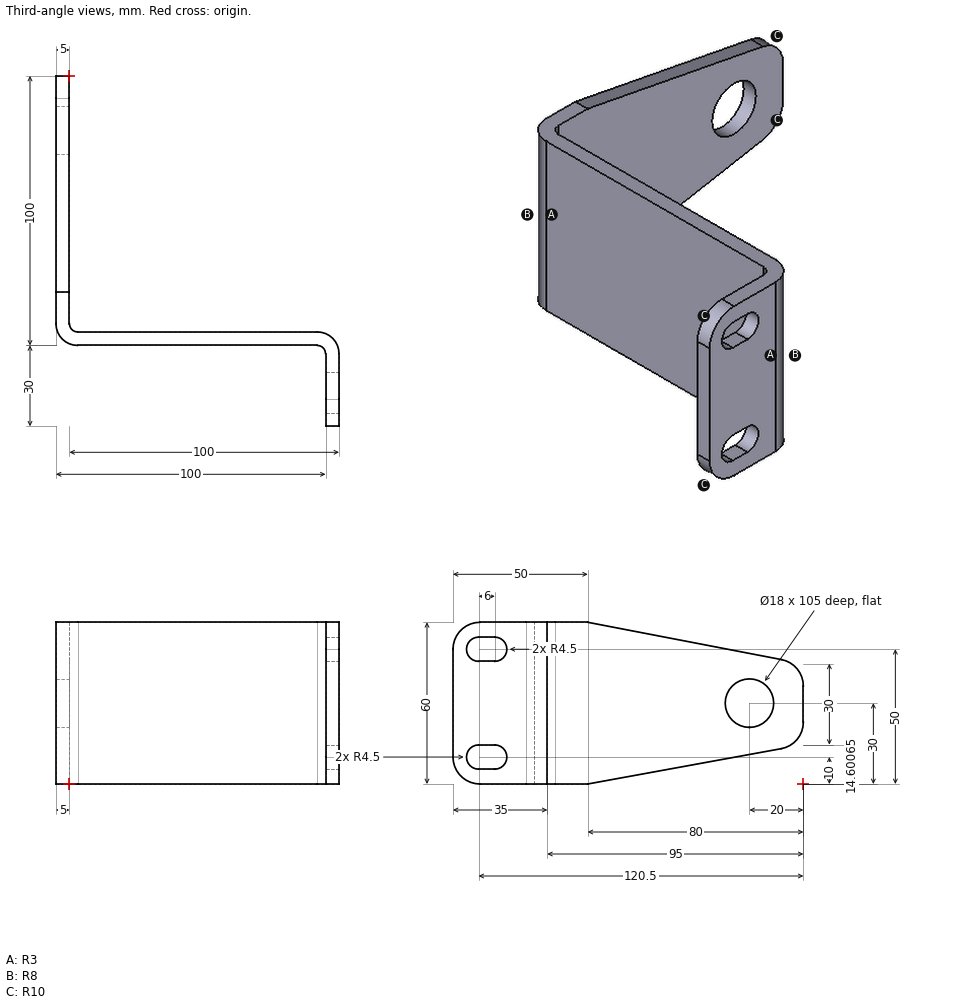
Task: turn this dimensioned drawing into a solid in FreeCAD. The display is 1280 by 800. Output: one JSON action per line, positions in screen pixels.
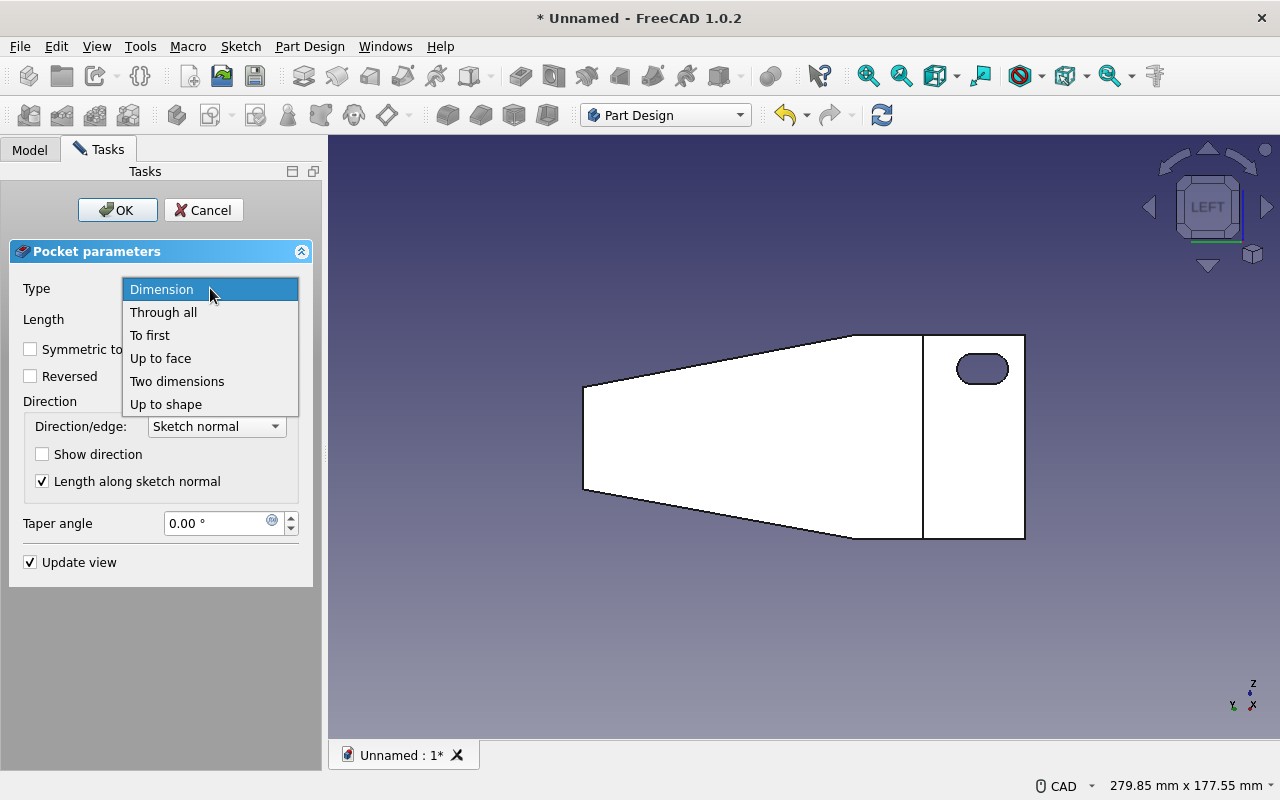
{"action": "left_click", "coordinate": [208, 312]}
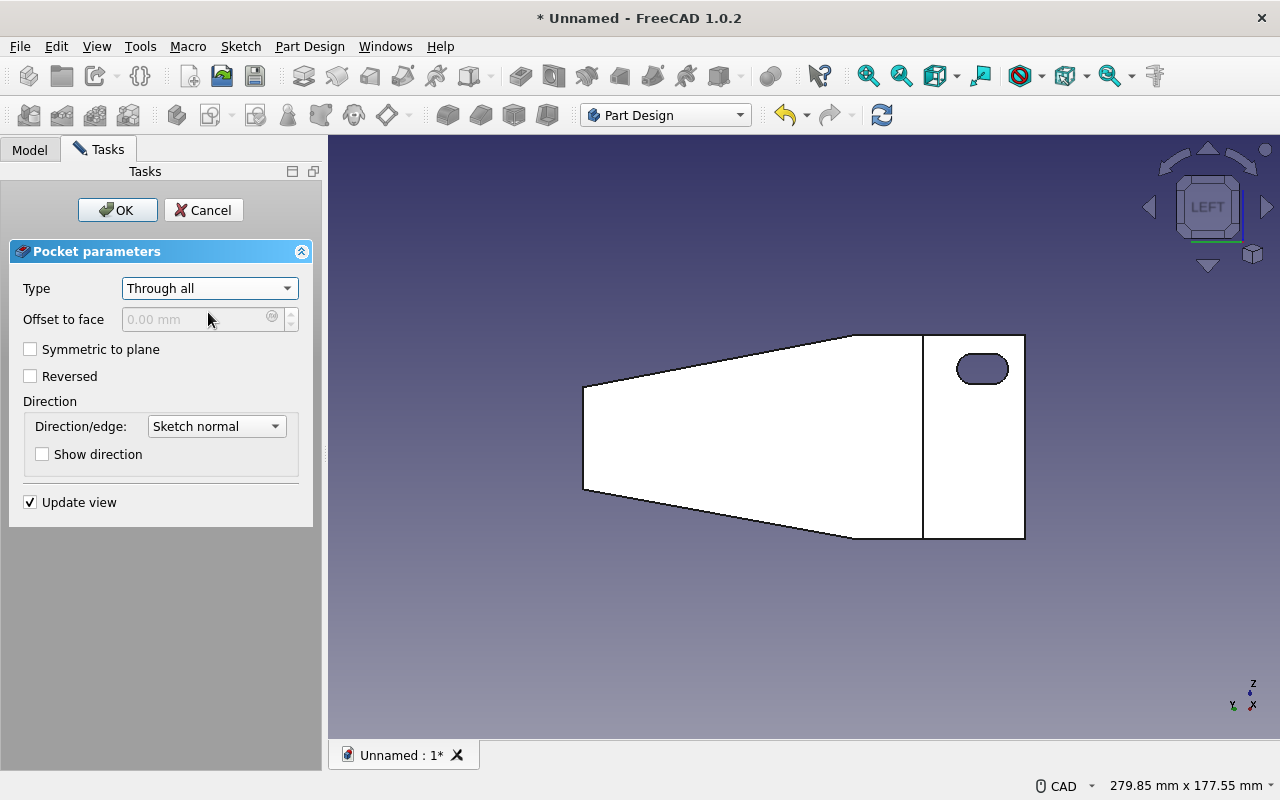
{"action": "left_click", "coordinate": [118, 210]}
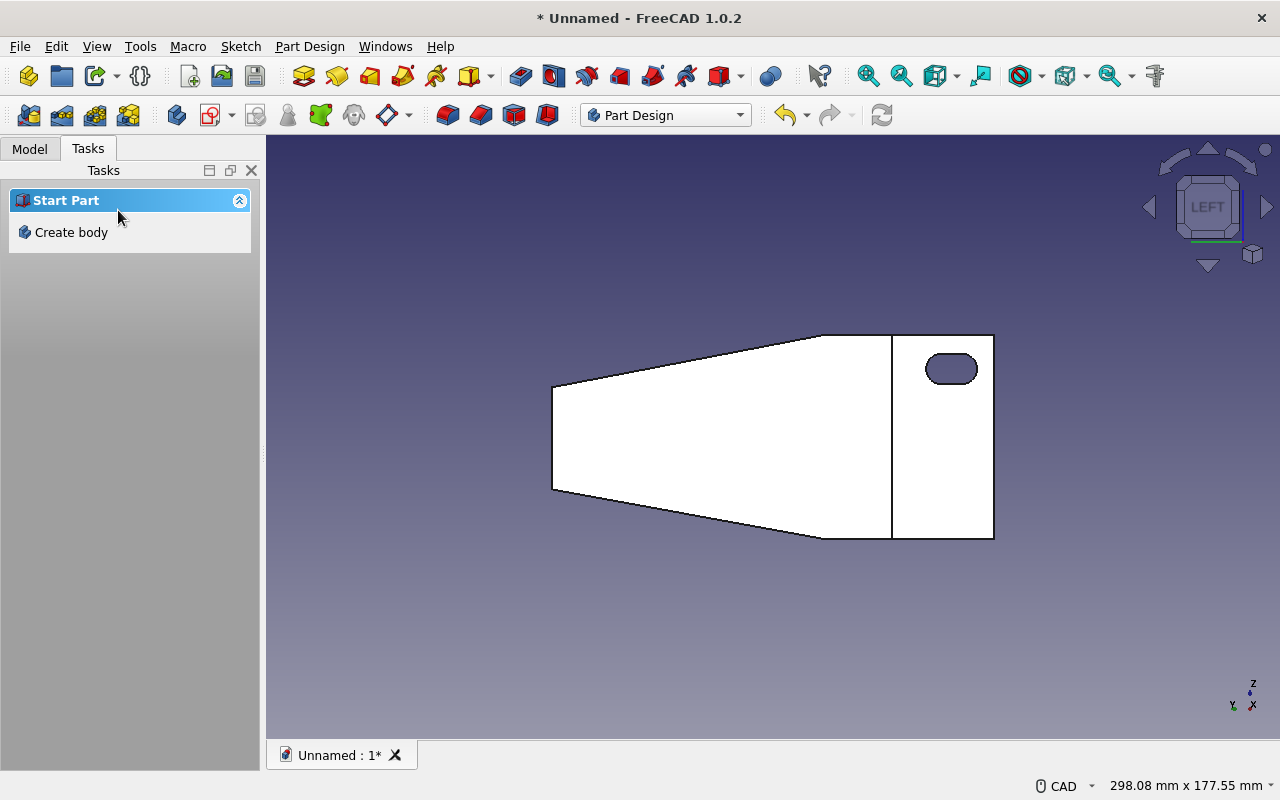
{"action": "left_click", "coordinate": [869, 76]}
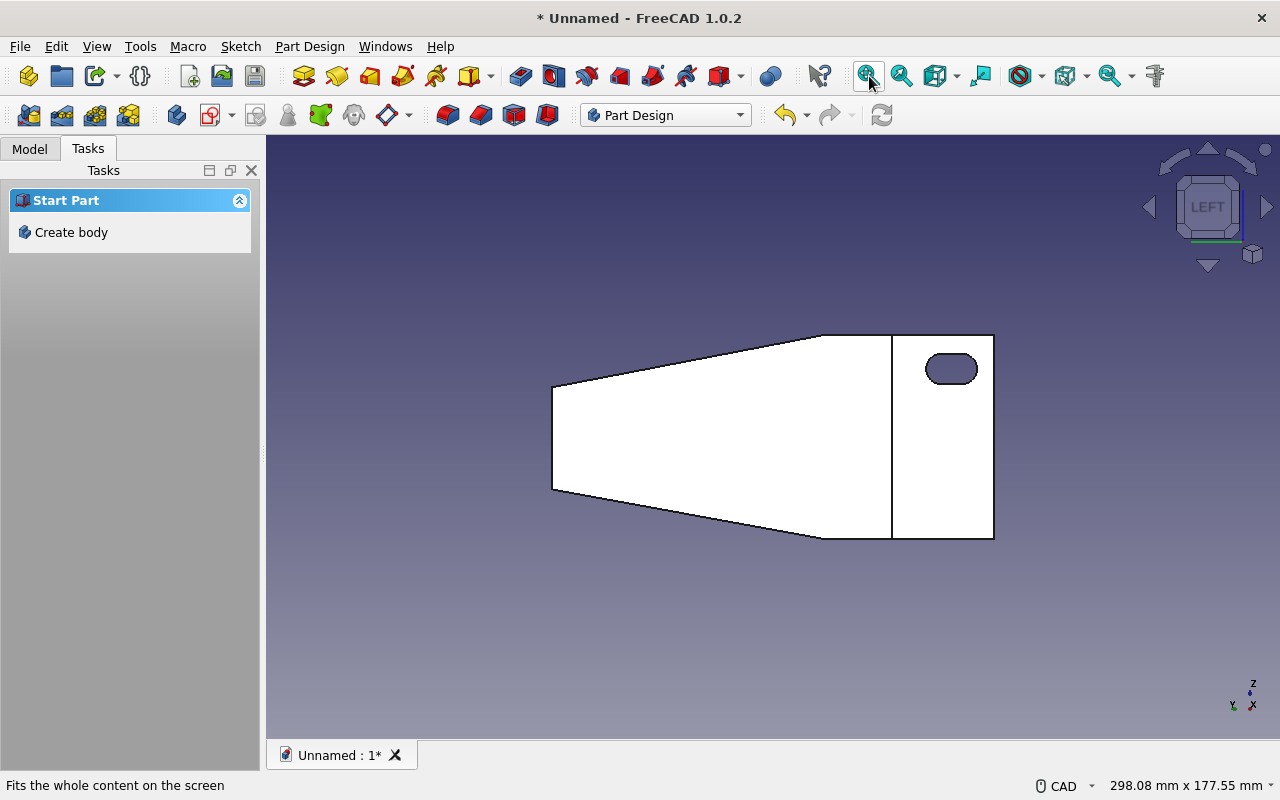
{"action": "key", "text": "0"}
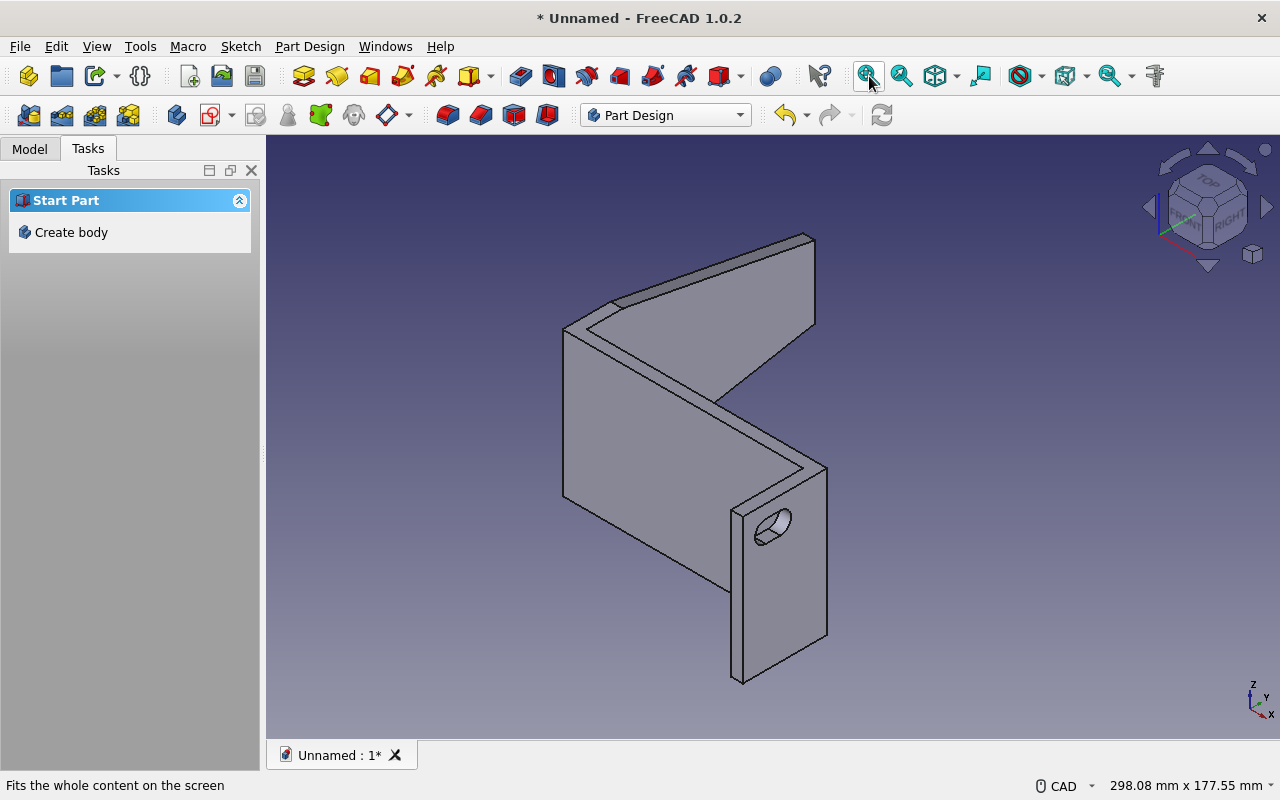
{"action": "left_click", "coordinate": [785, 599]}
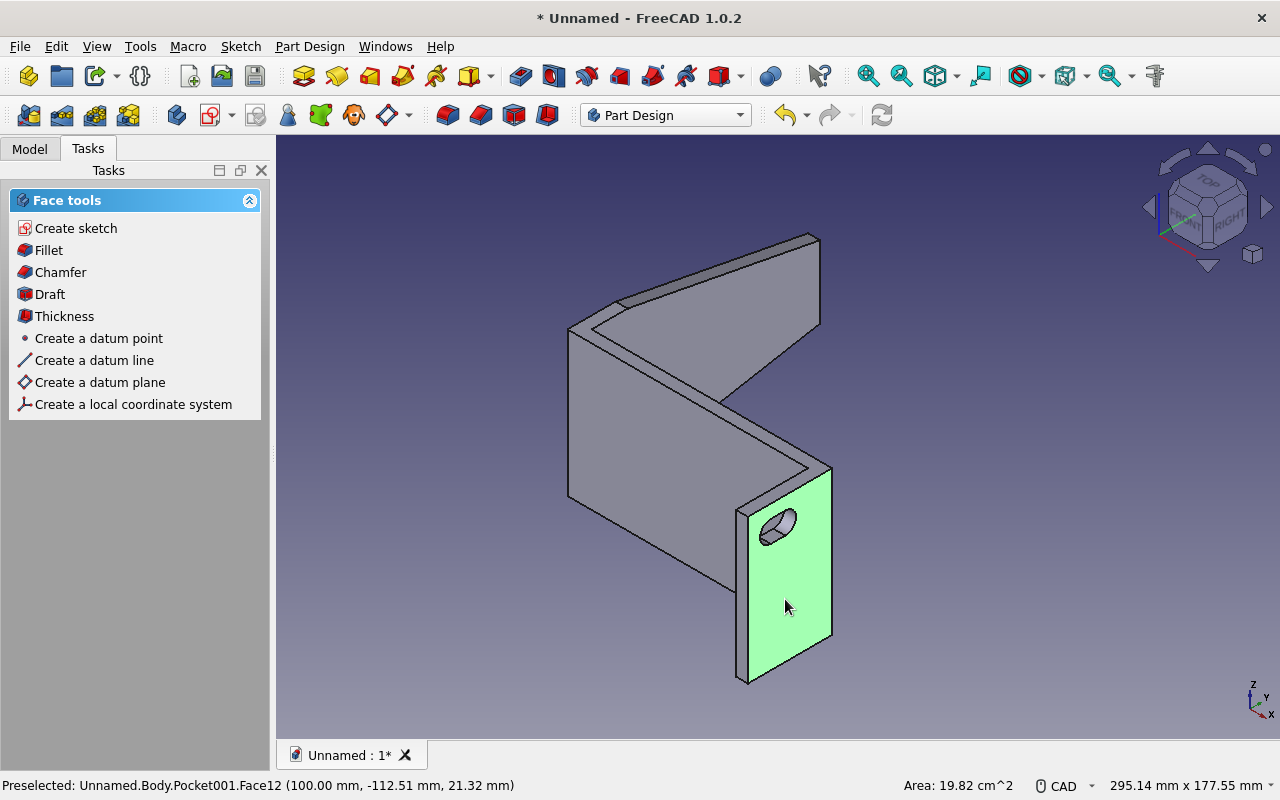
{"action": "left_click", "coordinate": [210, 116]}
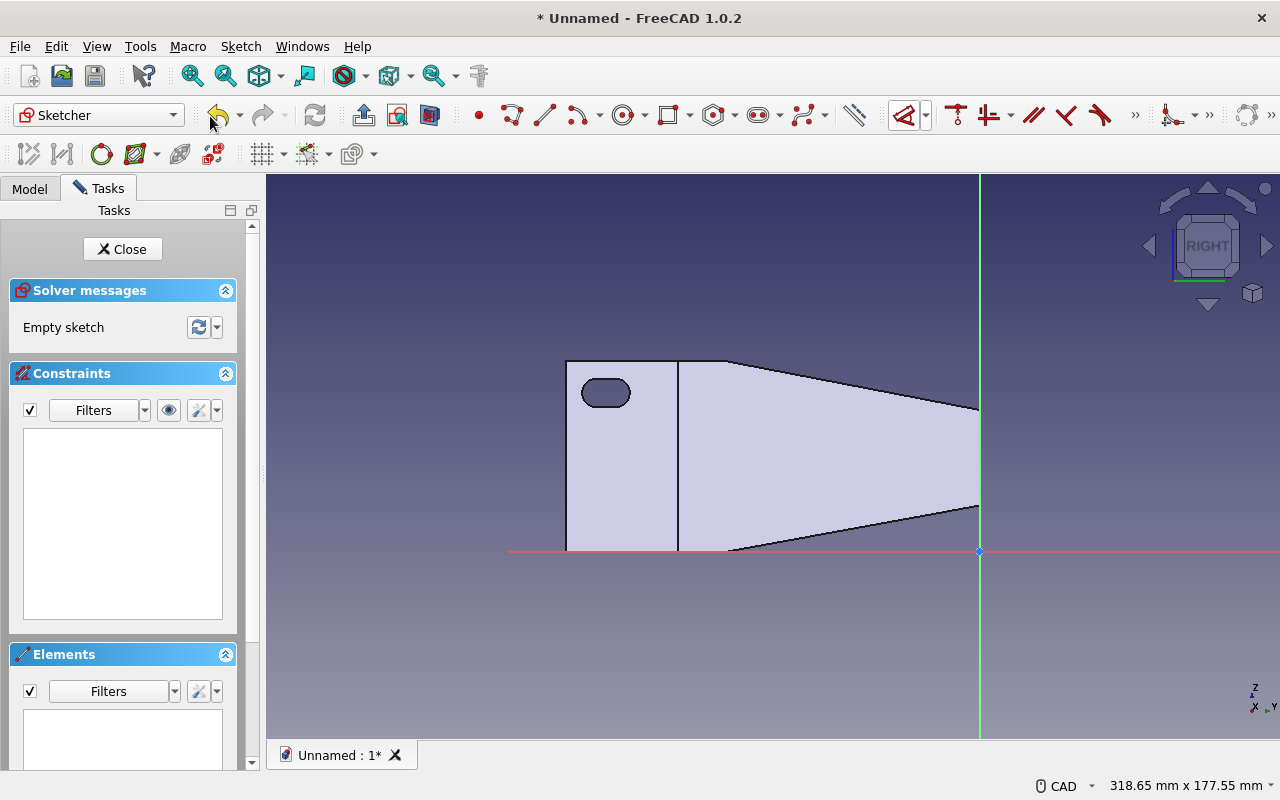
{"action": "scroll", "coordinate": [596, 526], "scroll_direction": "up", "scroll_amount": 12}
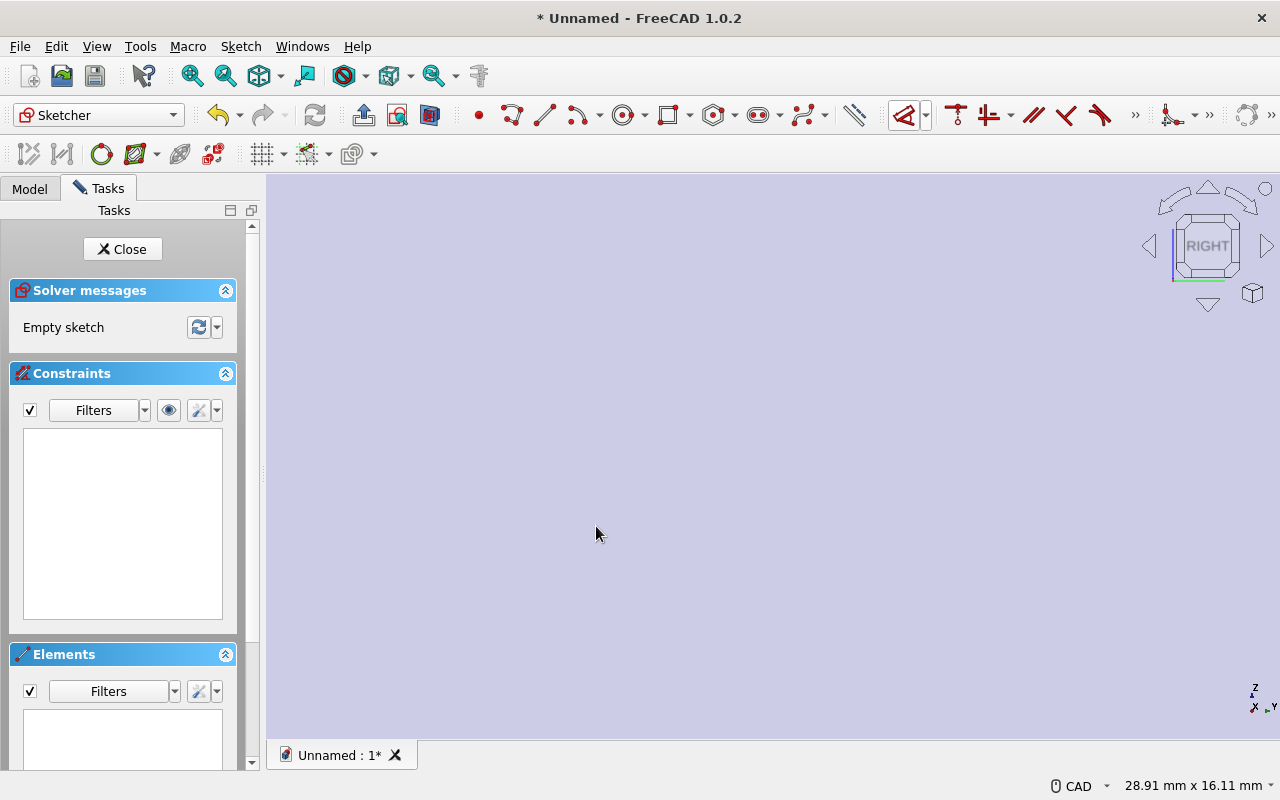
{"action": "left_click", "coordinate": [758, 116]}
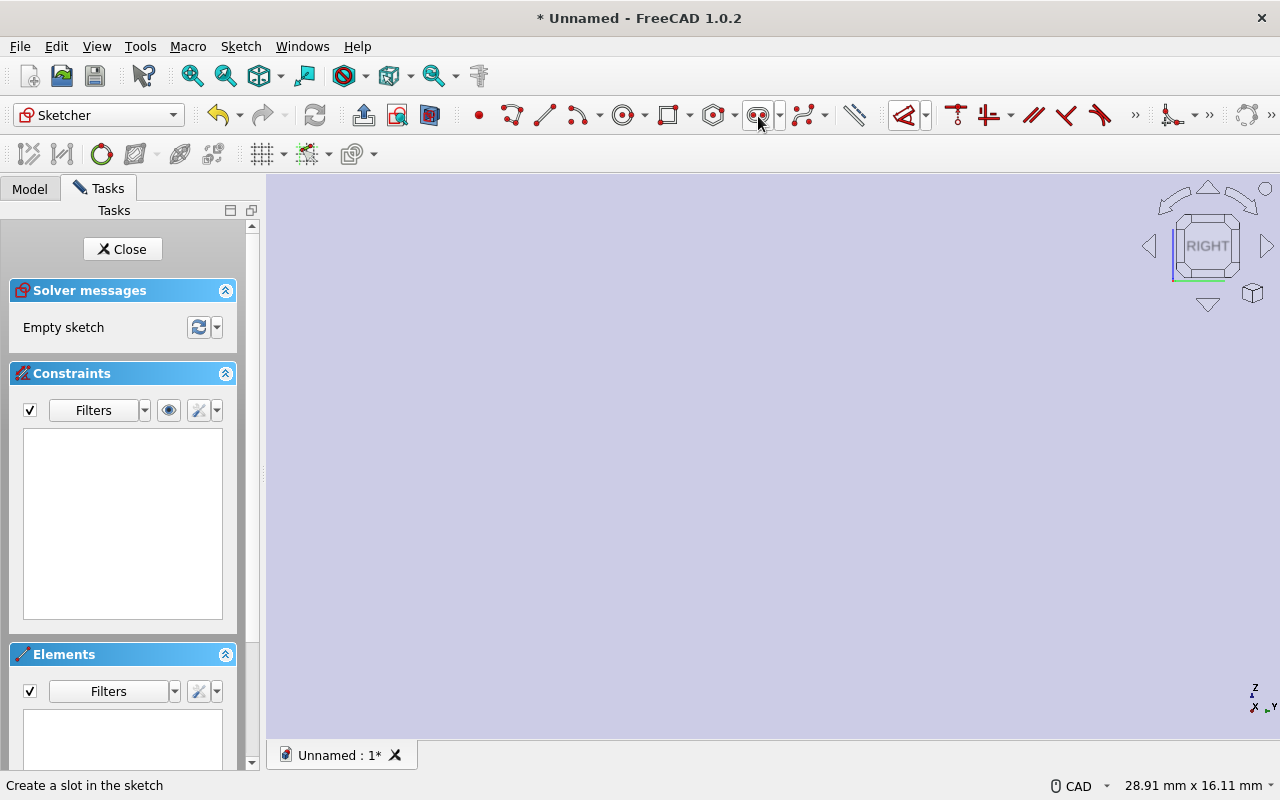
{"action": "left_click", "coordinate": [597, 455]}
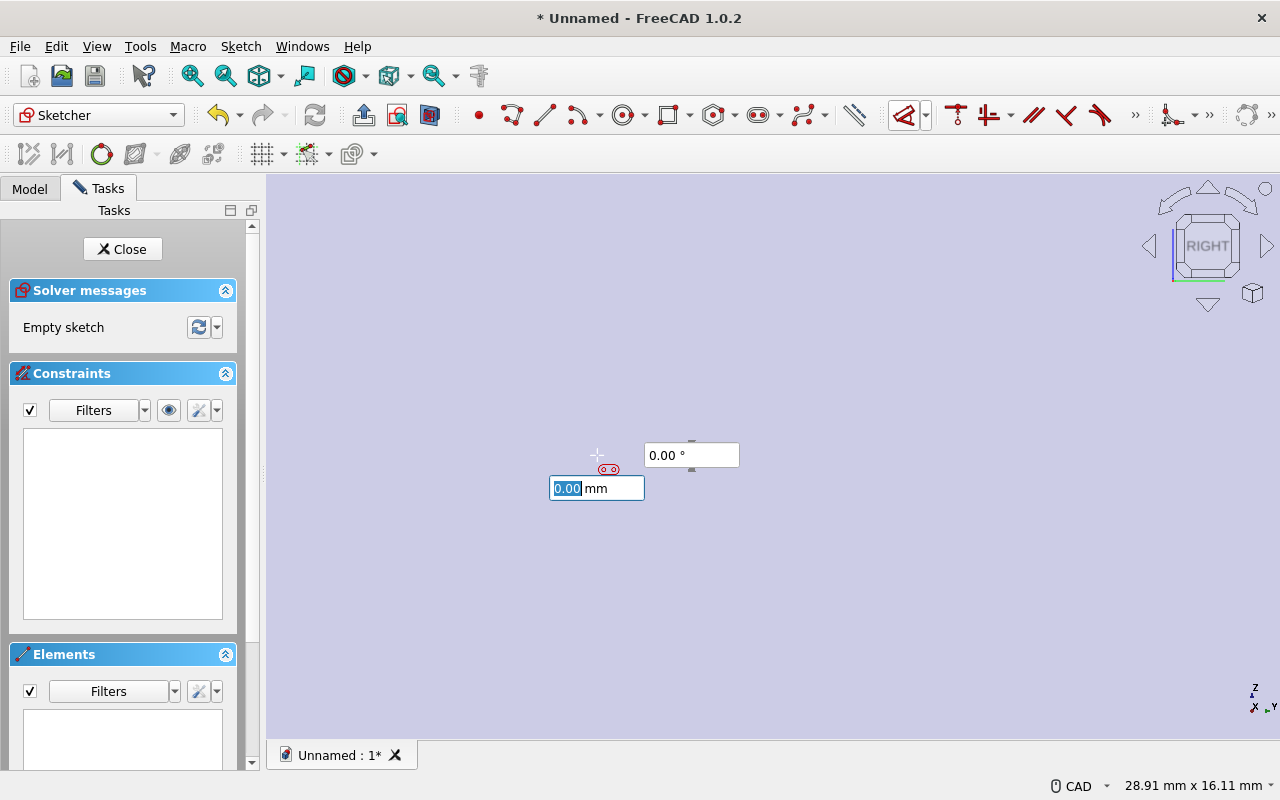
{"action": "left_click", "coordinate": [808, 455]}